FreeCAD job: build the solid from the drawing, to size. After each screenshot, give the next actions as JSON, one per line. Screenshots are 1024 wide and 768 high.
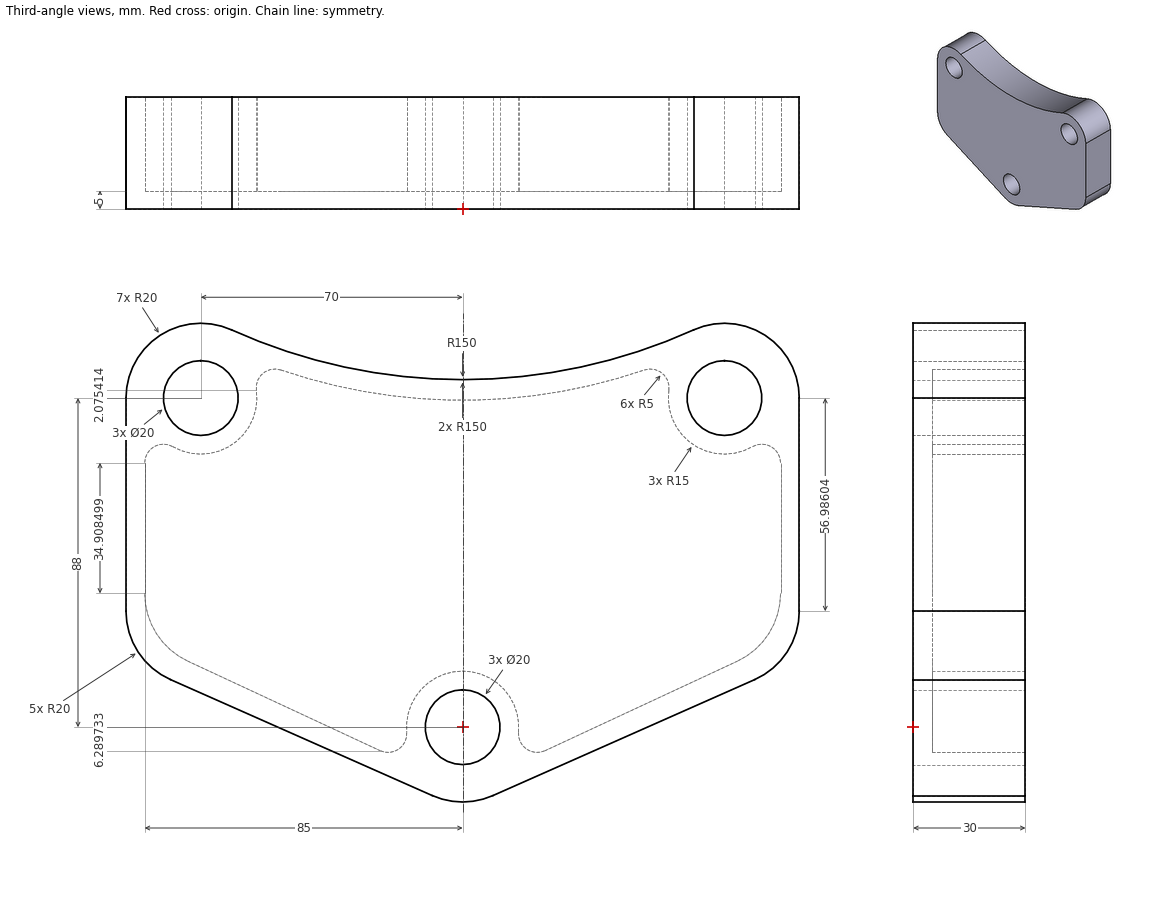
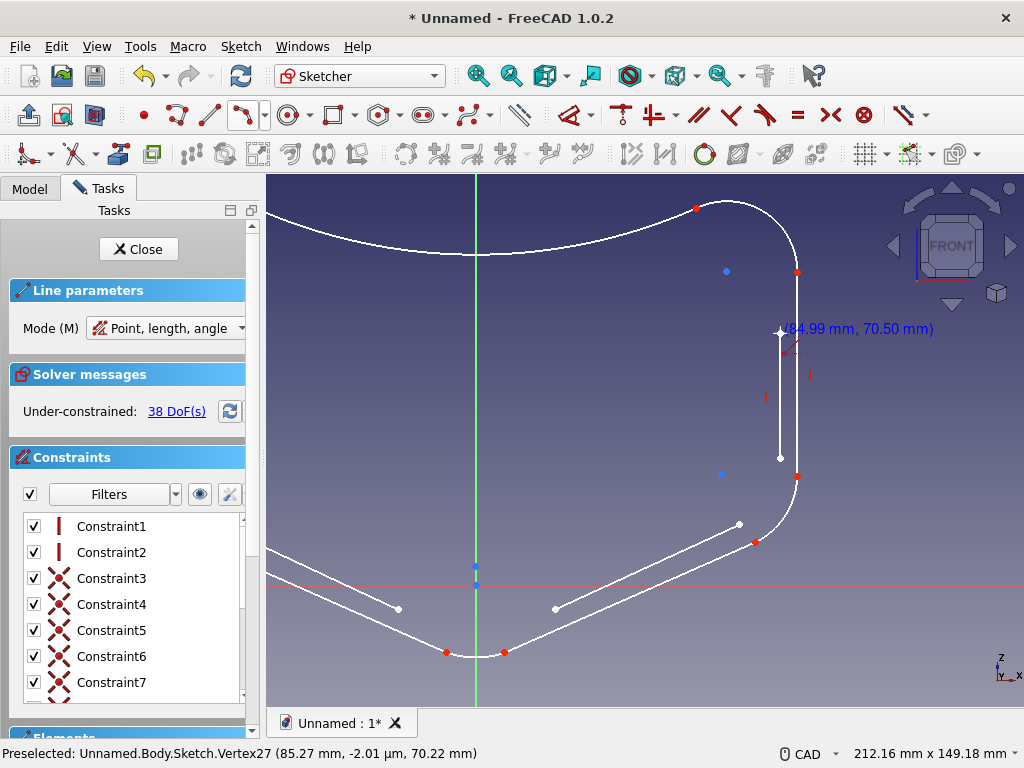
{"action": "left_click", "coordinate": [242, 116]}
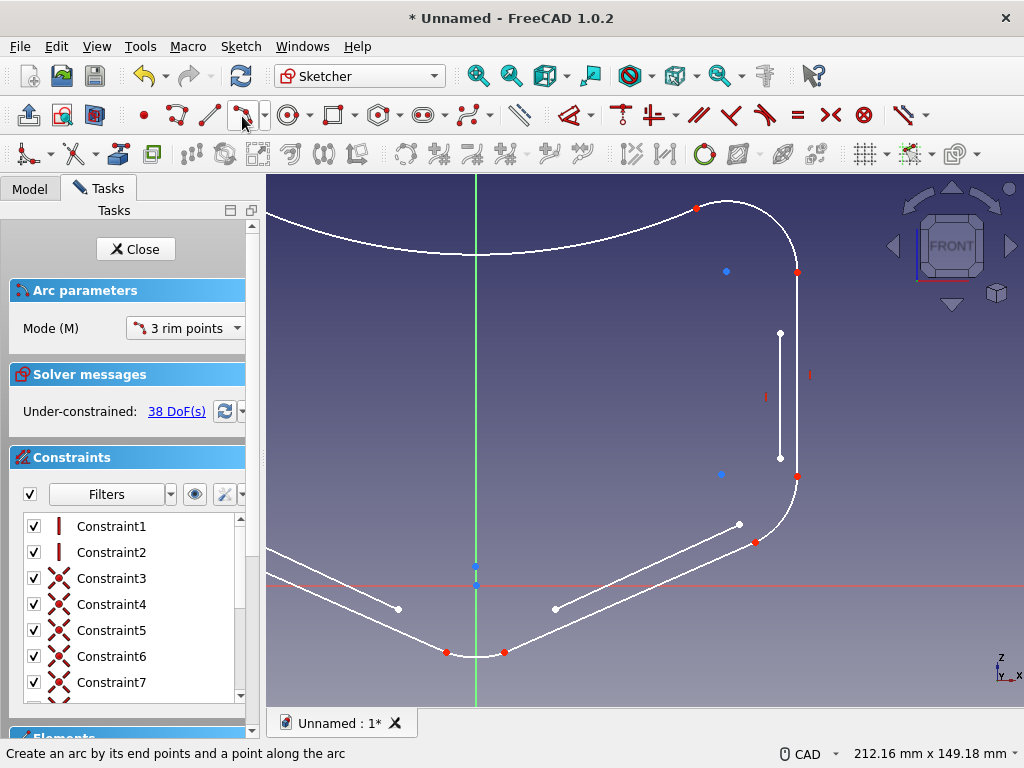
{"action": "scroll", "coordinate": [780, 458], "scroll_direction": "down", "scroll_amount": 2}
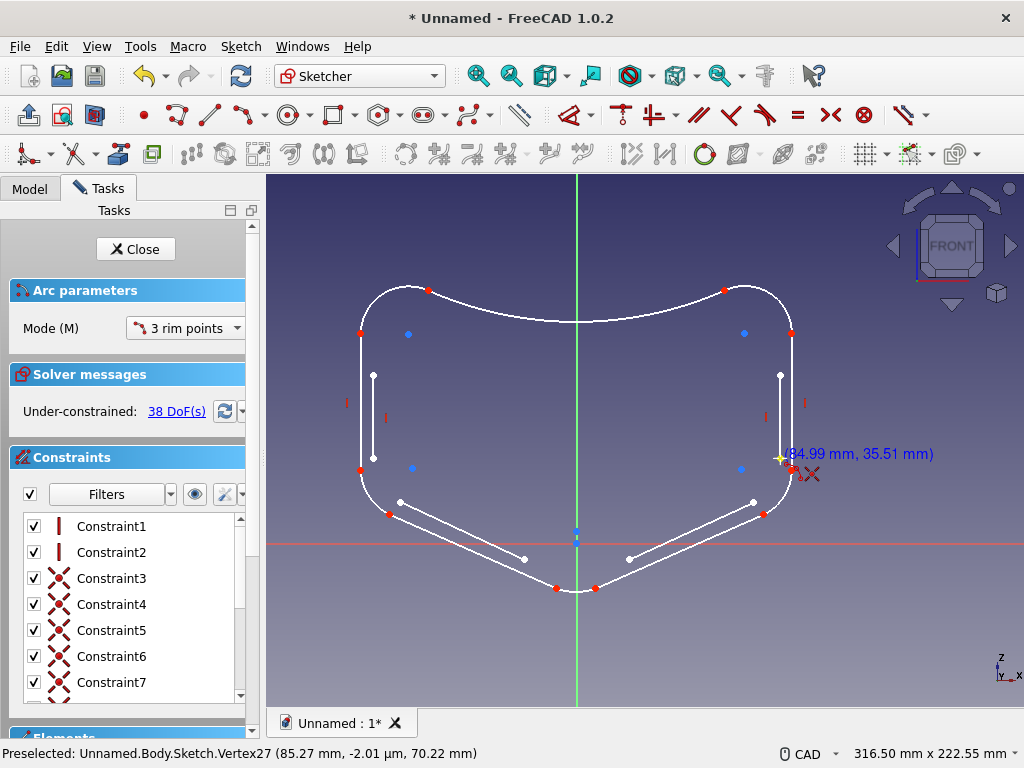
{"action": "scroll", "coordinate": [373, 458], "scroll_direction": "up", "scroll_amount": 2}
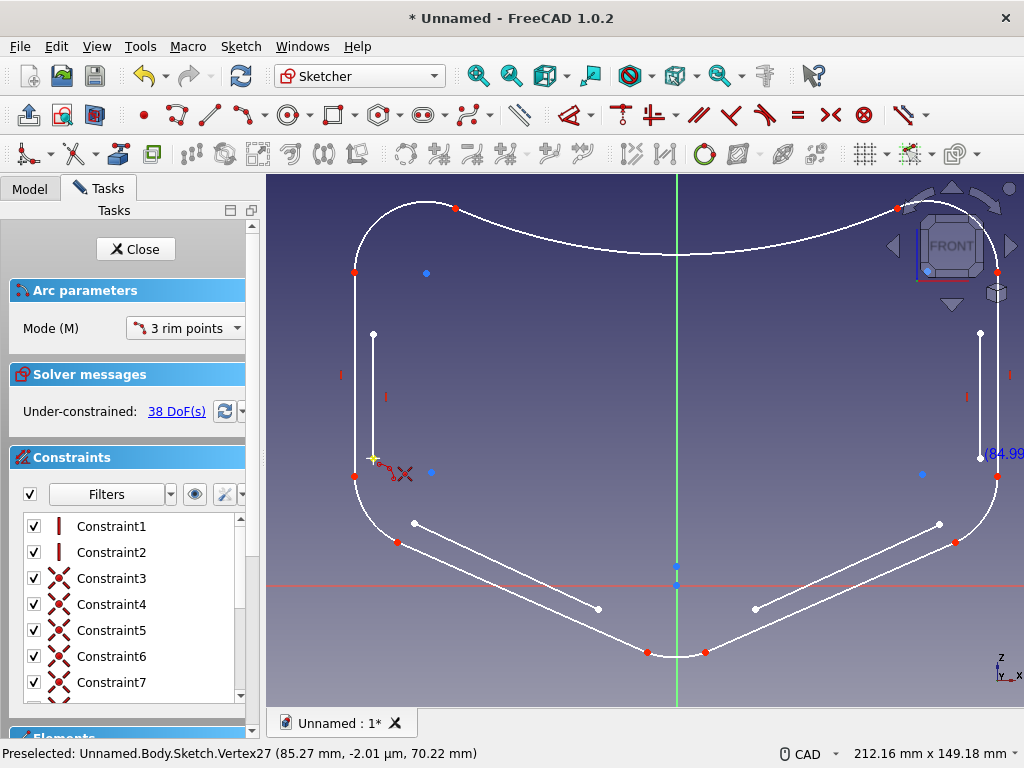
{"action": "left_click", "coordinate": [373, 459]}
{"action": "left_click", "coordinate": [414, 524]}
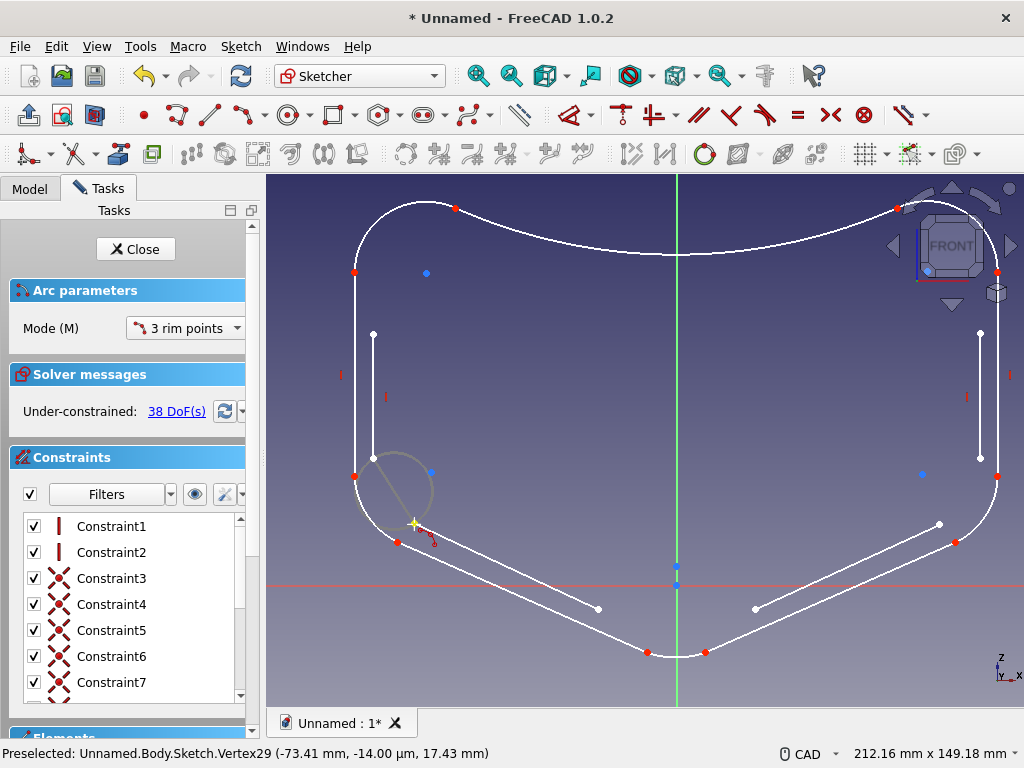
{"action": "scroll", "coordinate": [384, 496], "scroll_direction": "up", "scroll_amount": 2}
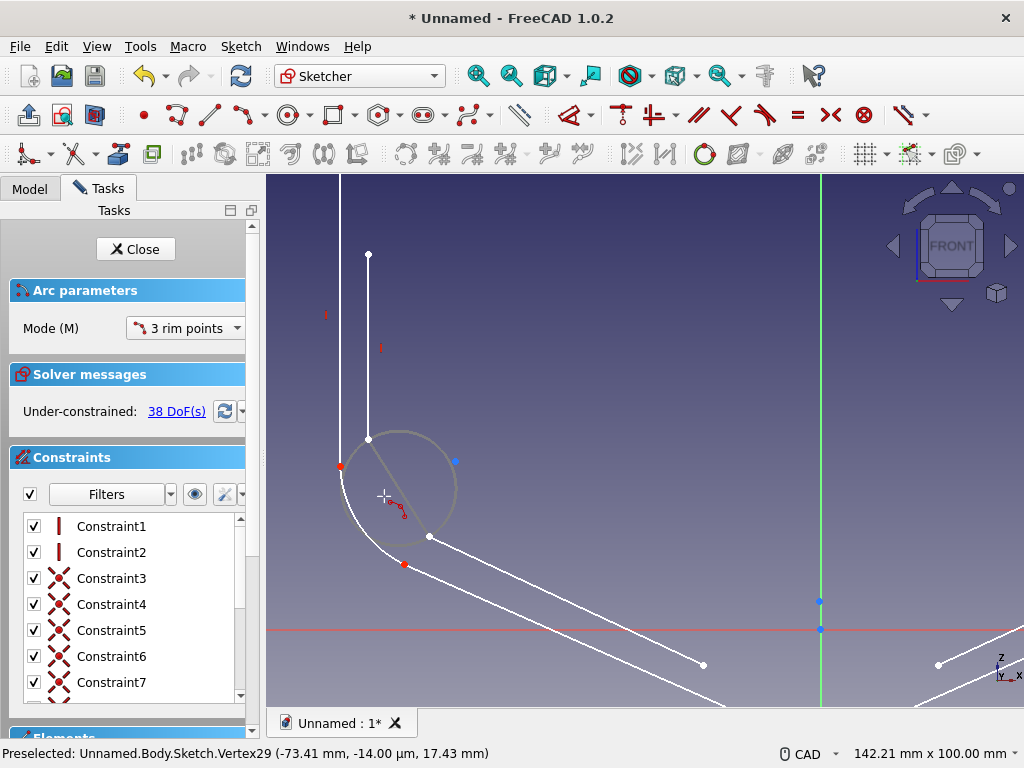
{"action": "left_click", "coordinate": [384, 496]}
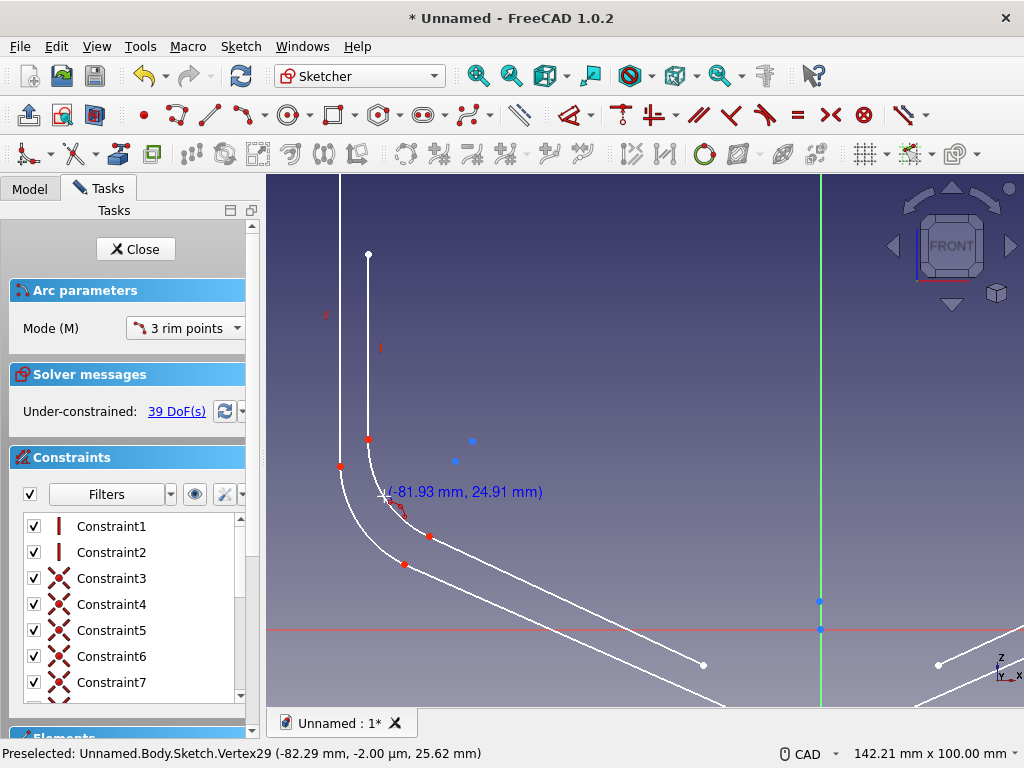
{"action": "left_click", "coordinate": [704, 665]}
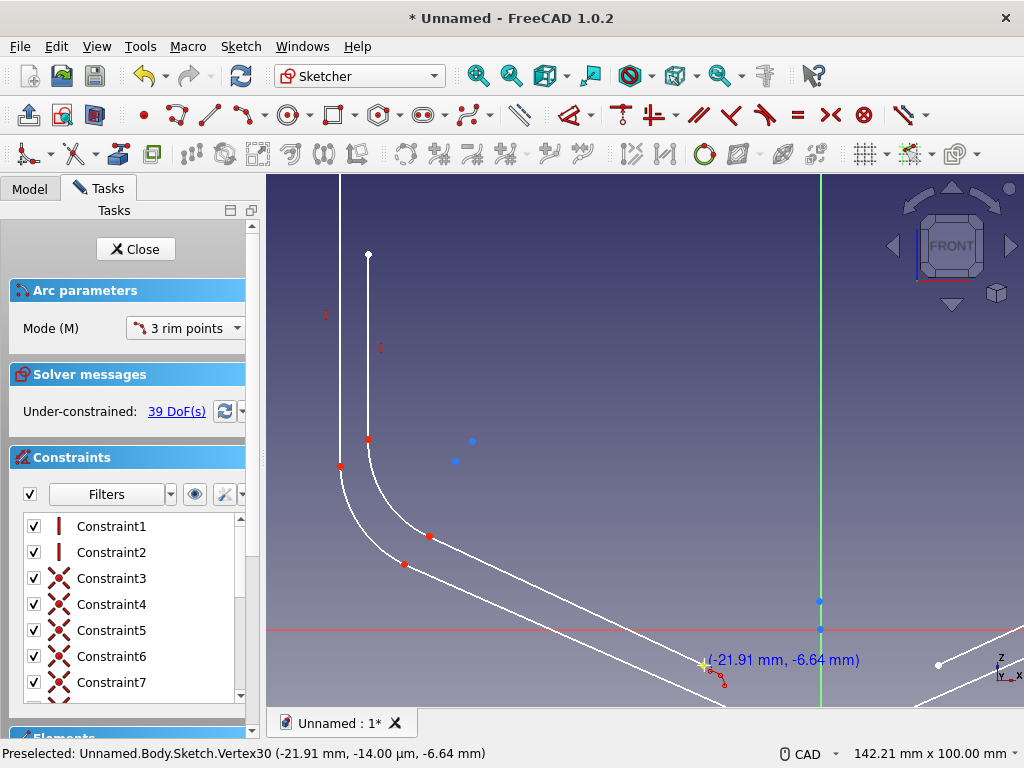
{"action": "scroll", "coordinate": [741, 637], "scroll_direction": "up", "scroll_amount": 5}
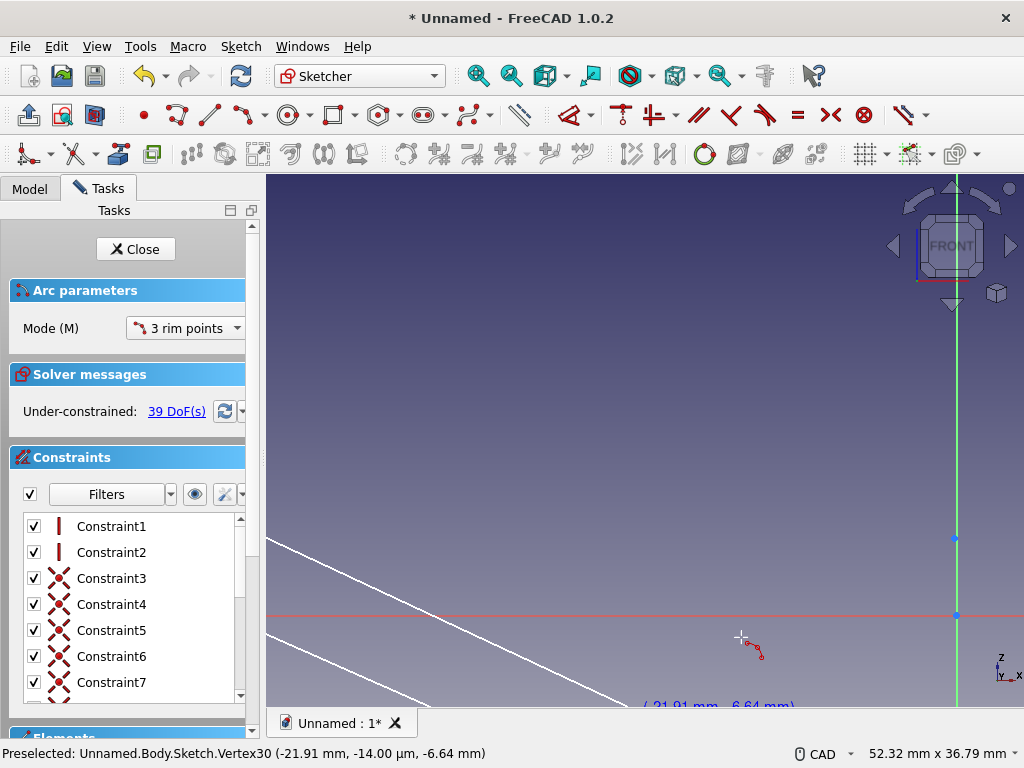
{"action": "left_click", "coordinate": [740, 635]}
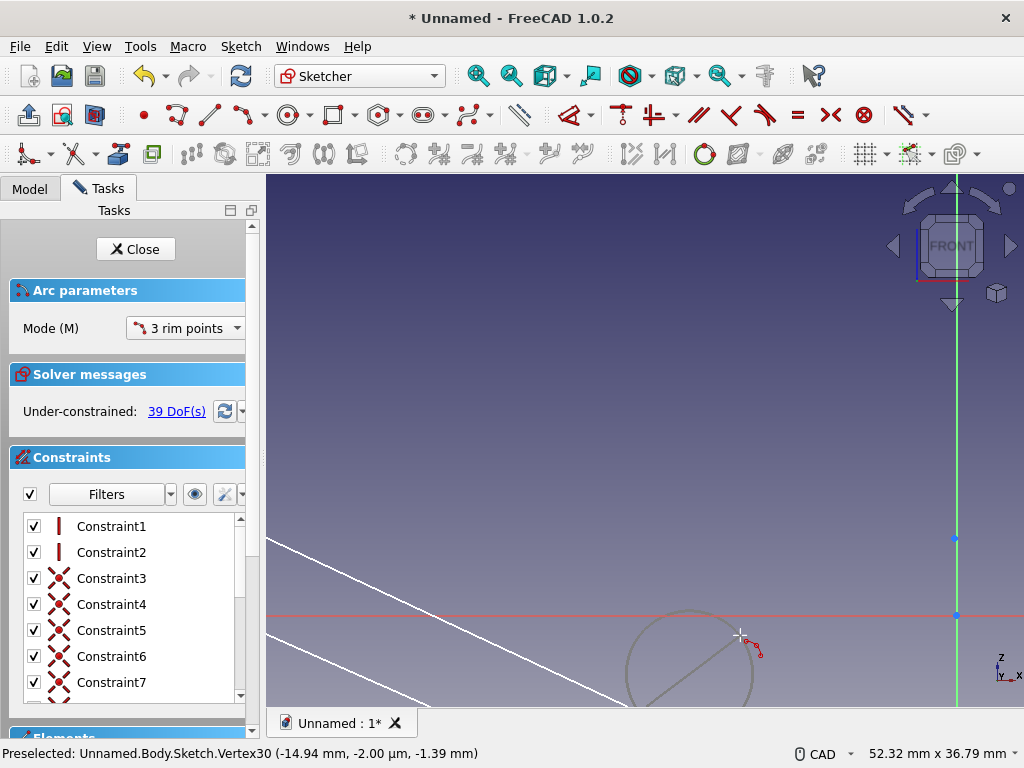
{"action": "scroll", "coordinate": [501, 529], "scroll_direction": "down", "scroll_amount": 9}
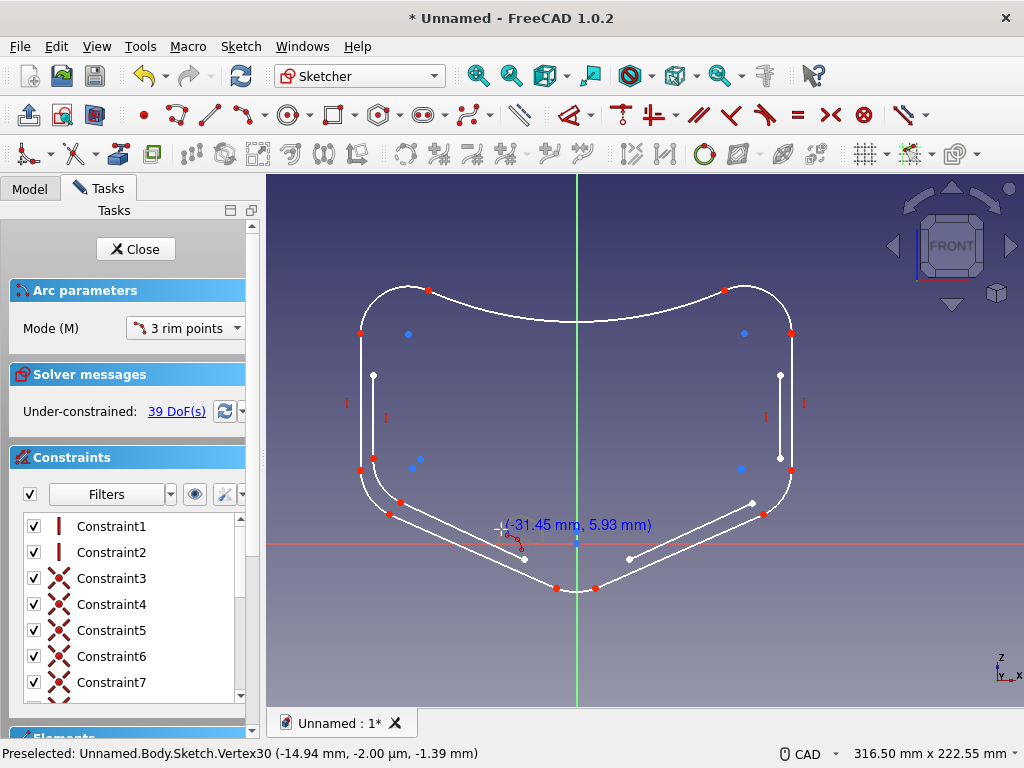
{"action": "scroll", "coordinate": [536, 558], "scroll_direction": "up", "scroll_amount": 5}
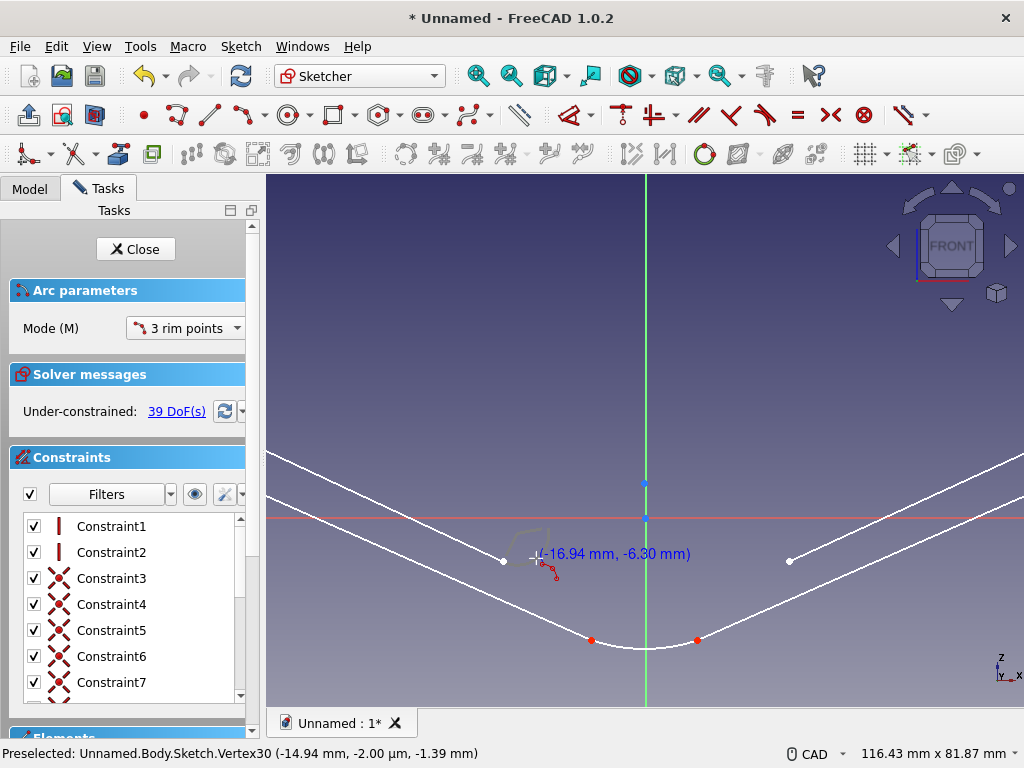
{"action": "left_click", "coordinate": [535, 557]}